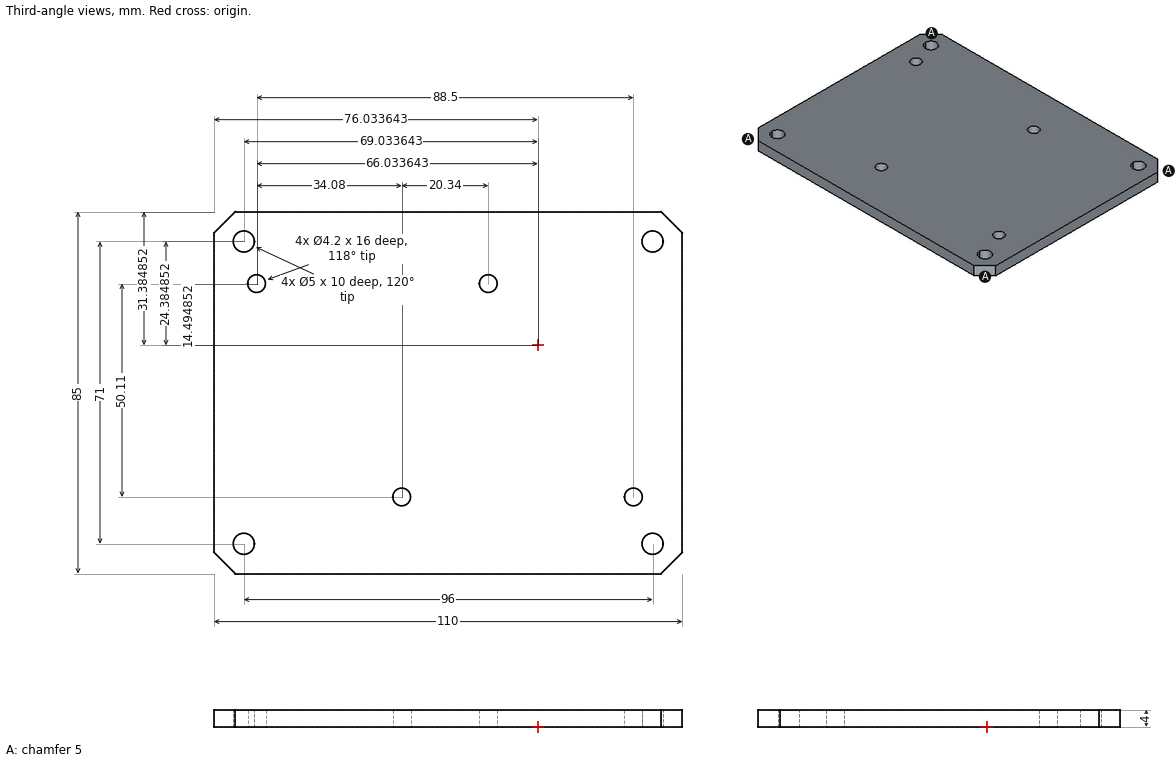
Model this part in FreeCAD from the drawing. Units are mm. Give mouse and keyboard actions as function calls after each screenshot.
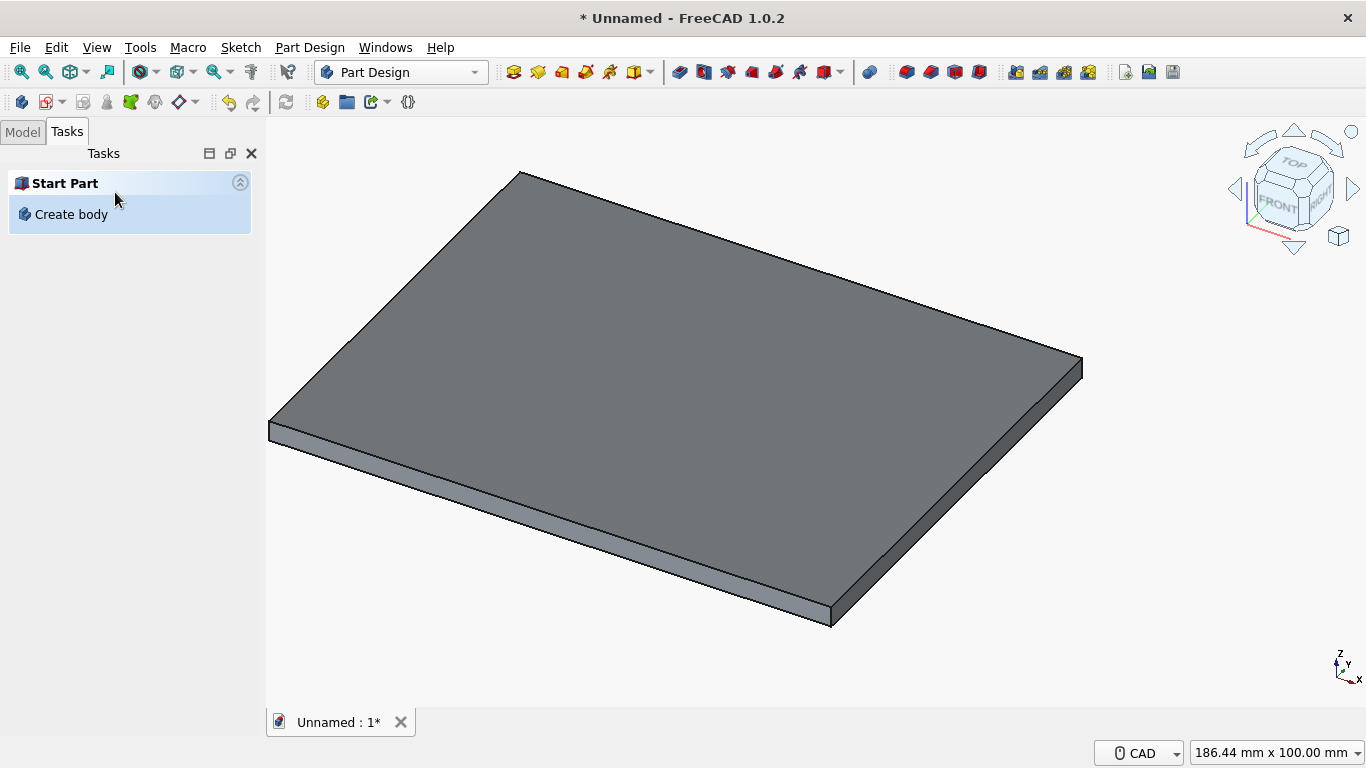
click(676, 389)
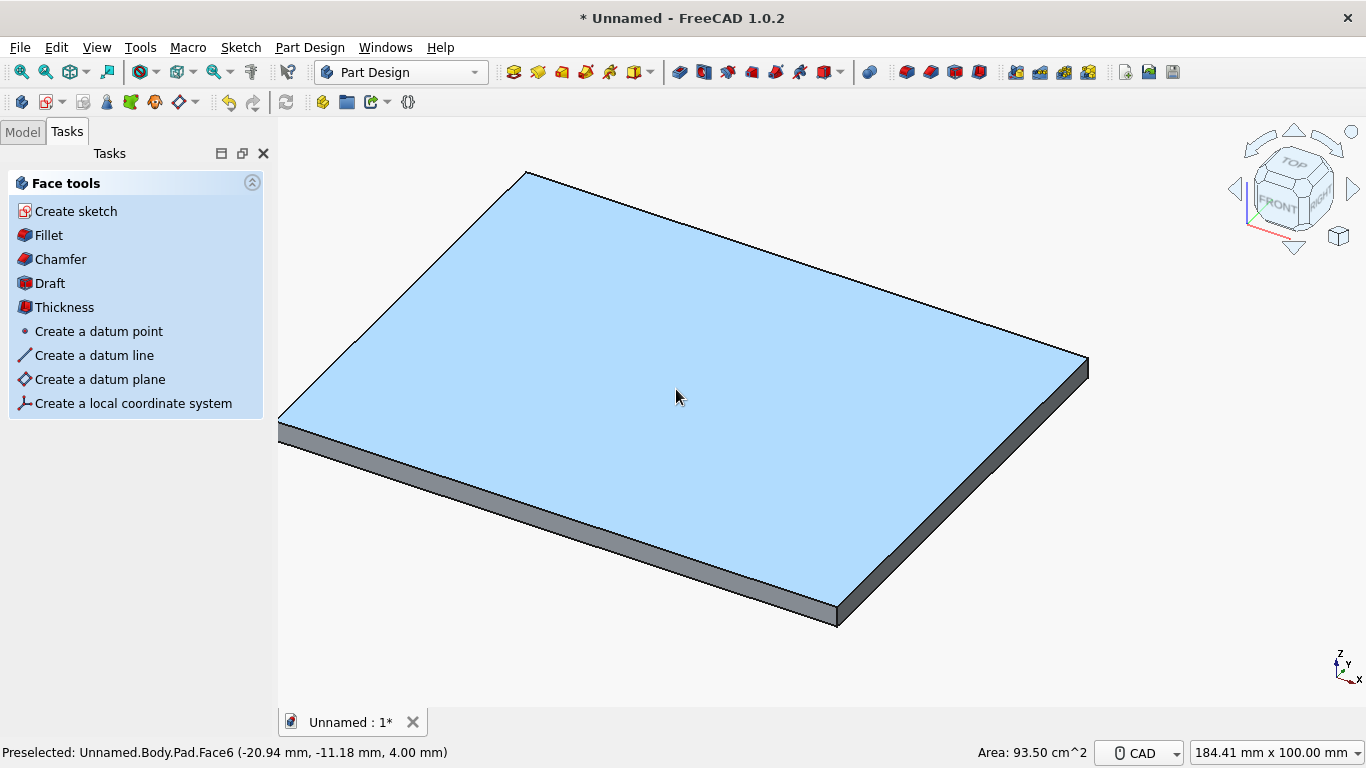
click(46, 102)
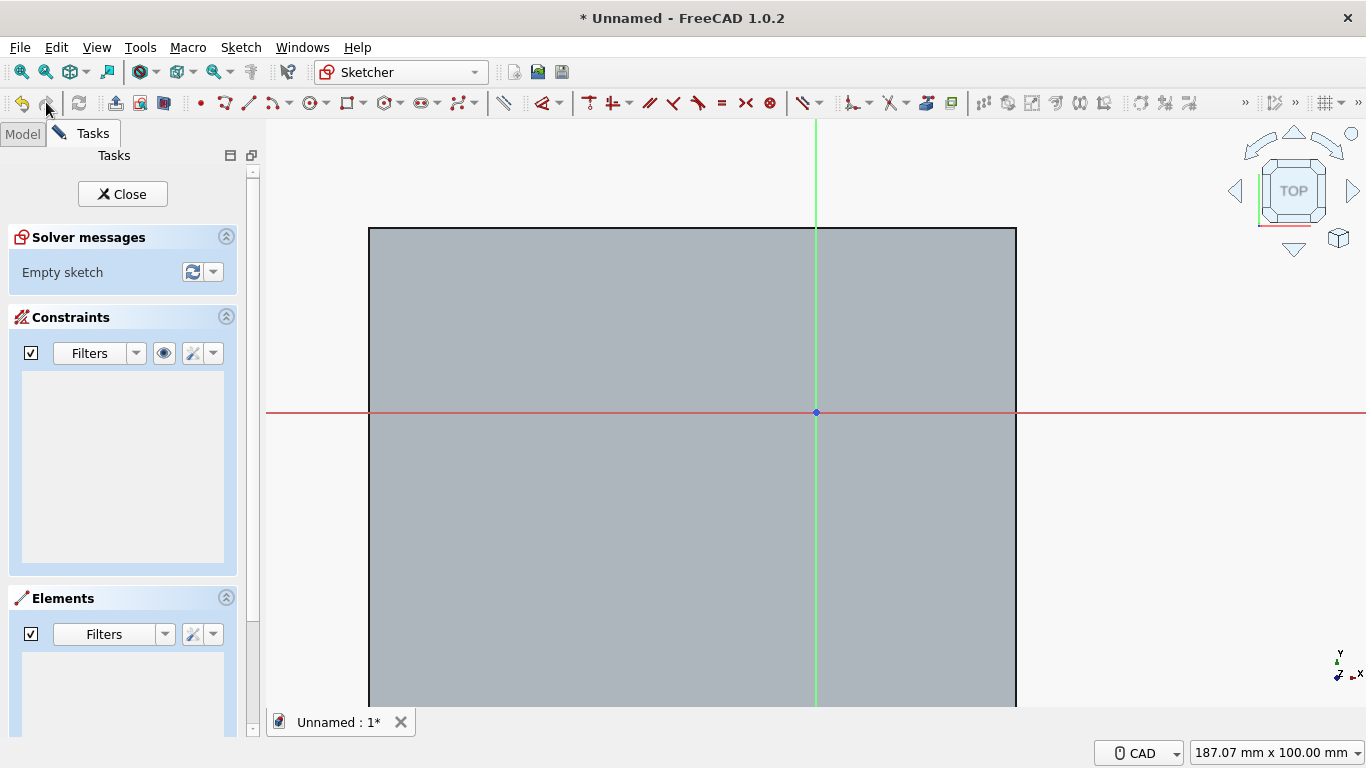
click(310, 104)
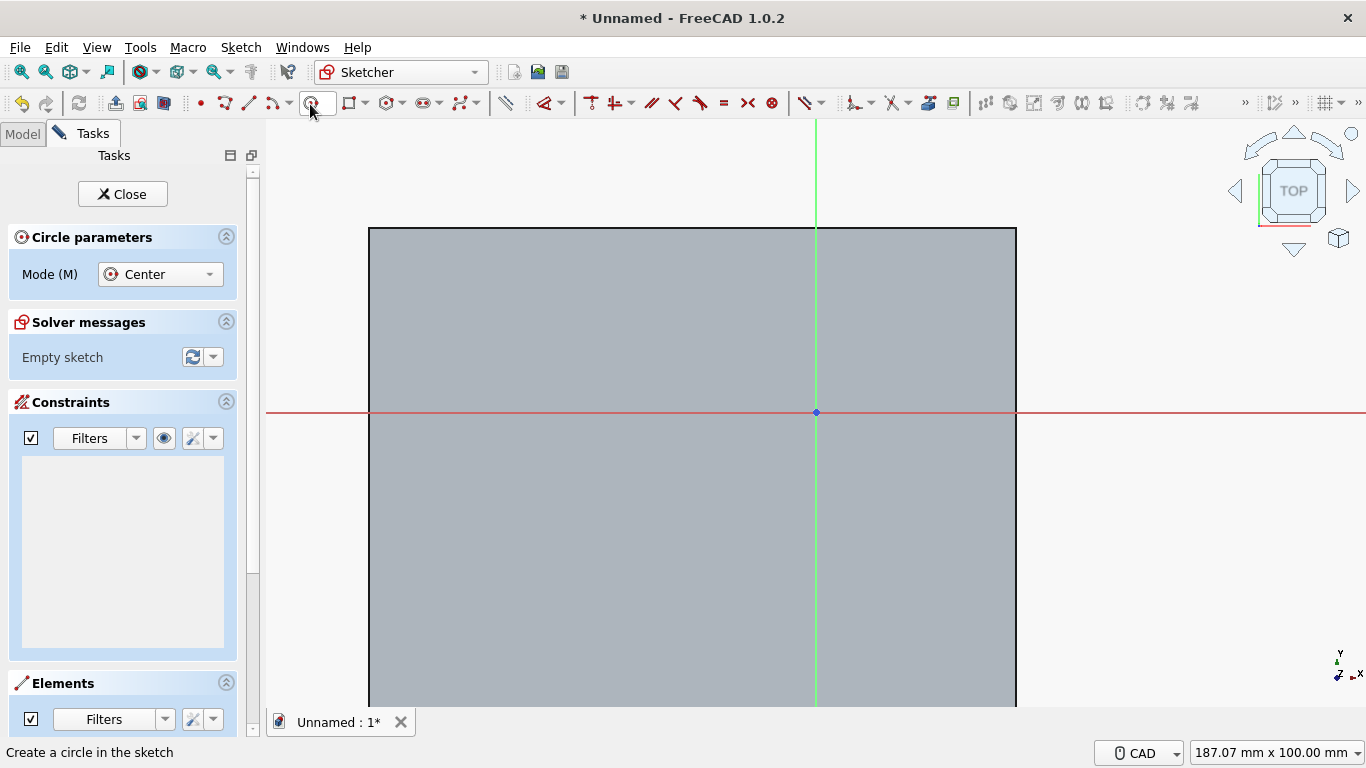
scroll(428, 328, up, 4)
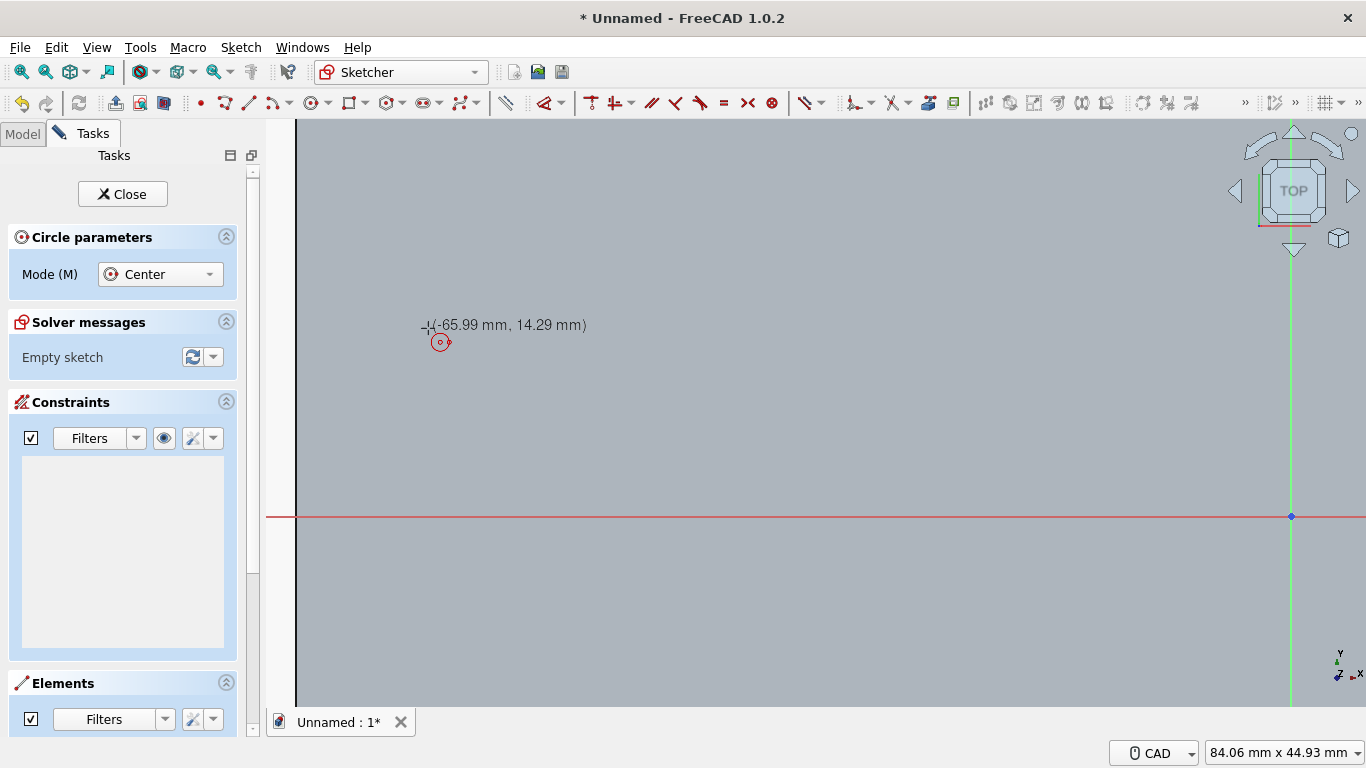
click(427, 327)
click(447, 308)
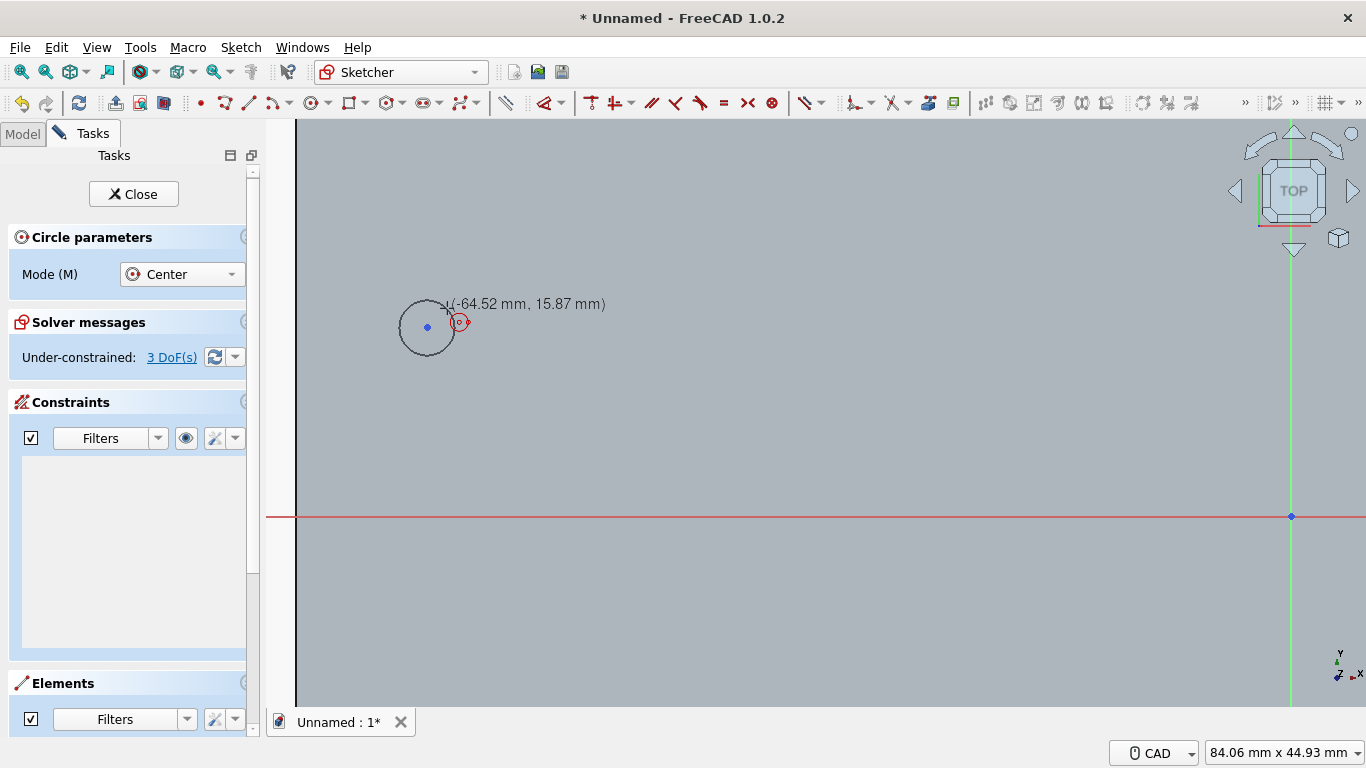
scroll(433, 147, down, 3)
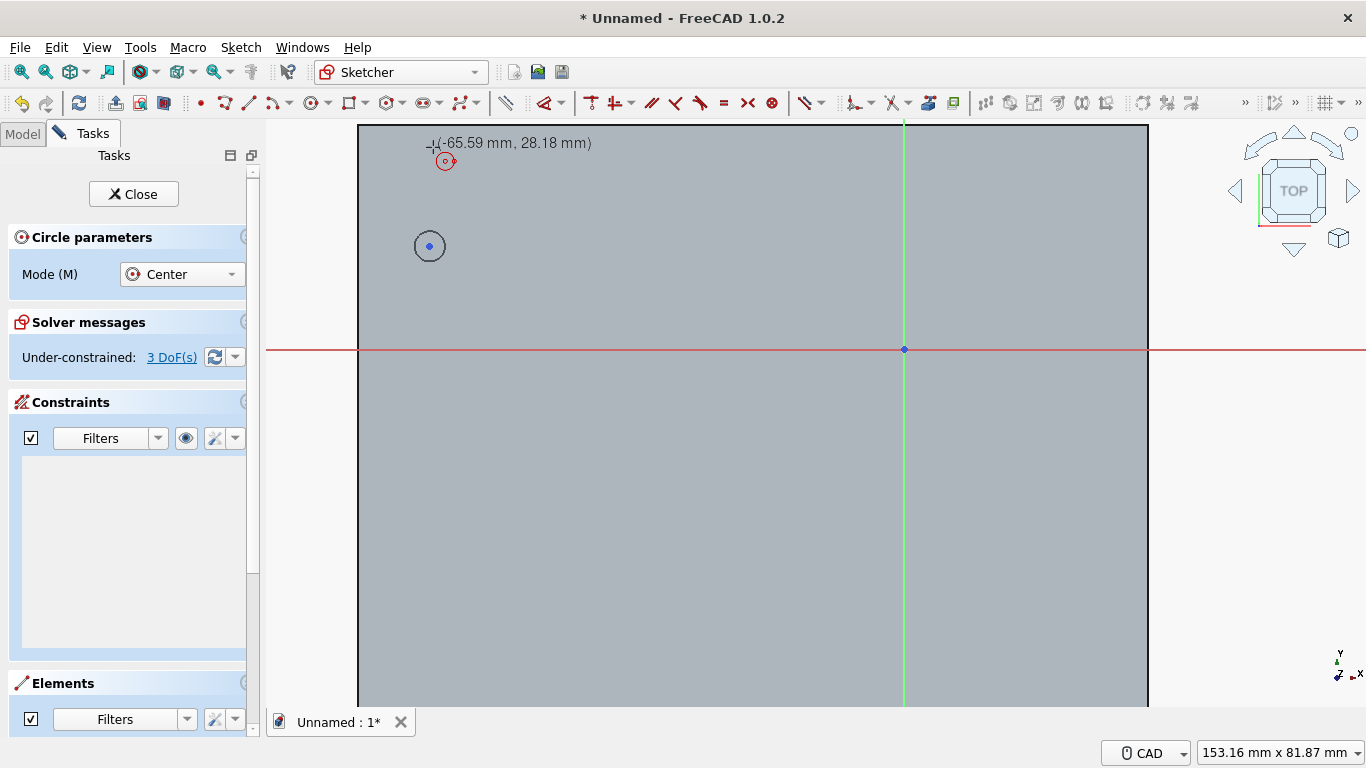
scroll(675, 606, up, 3)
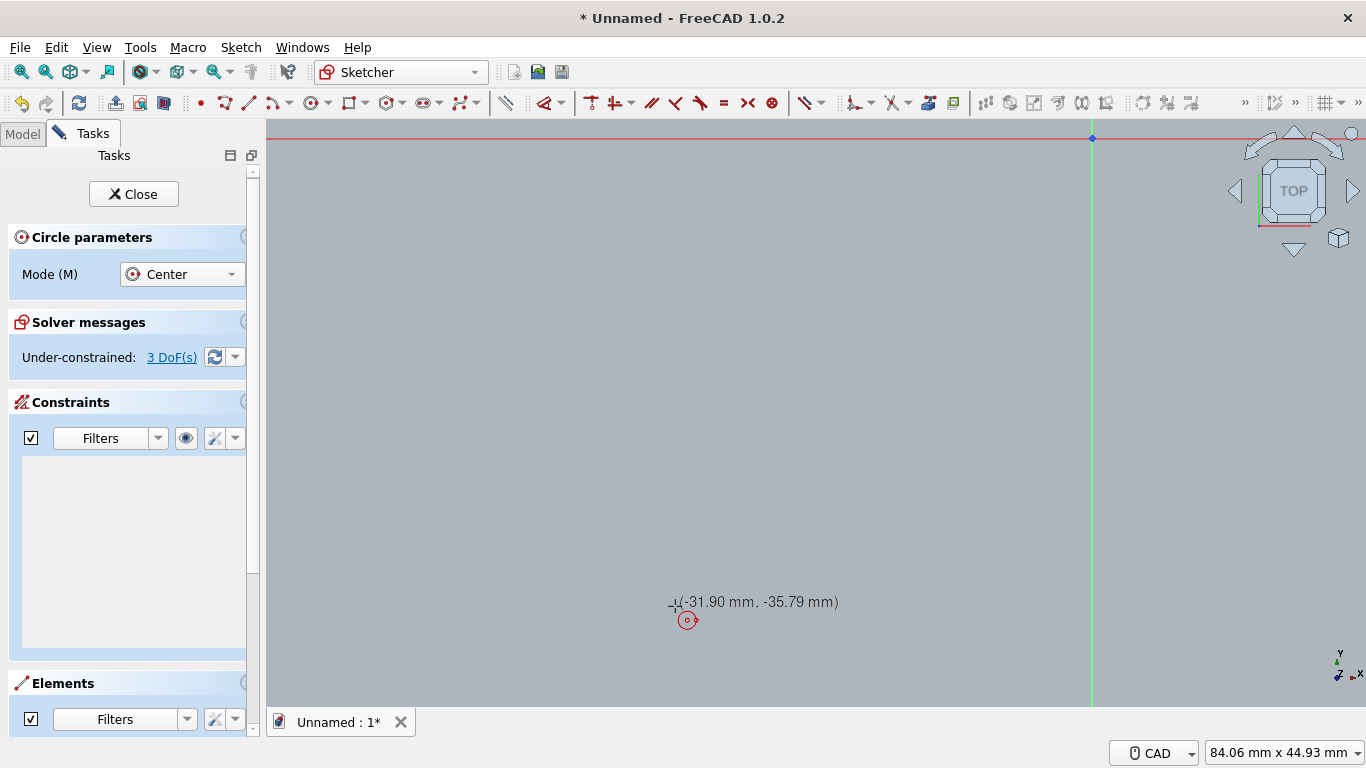
click(674, 605)
click(693, 585)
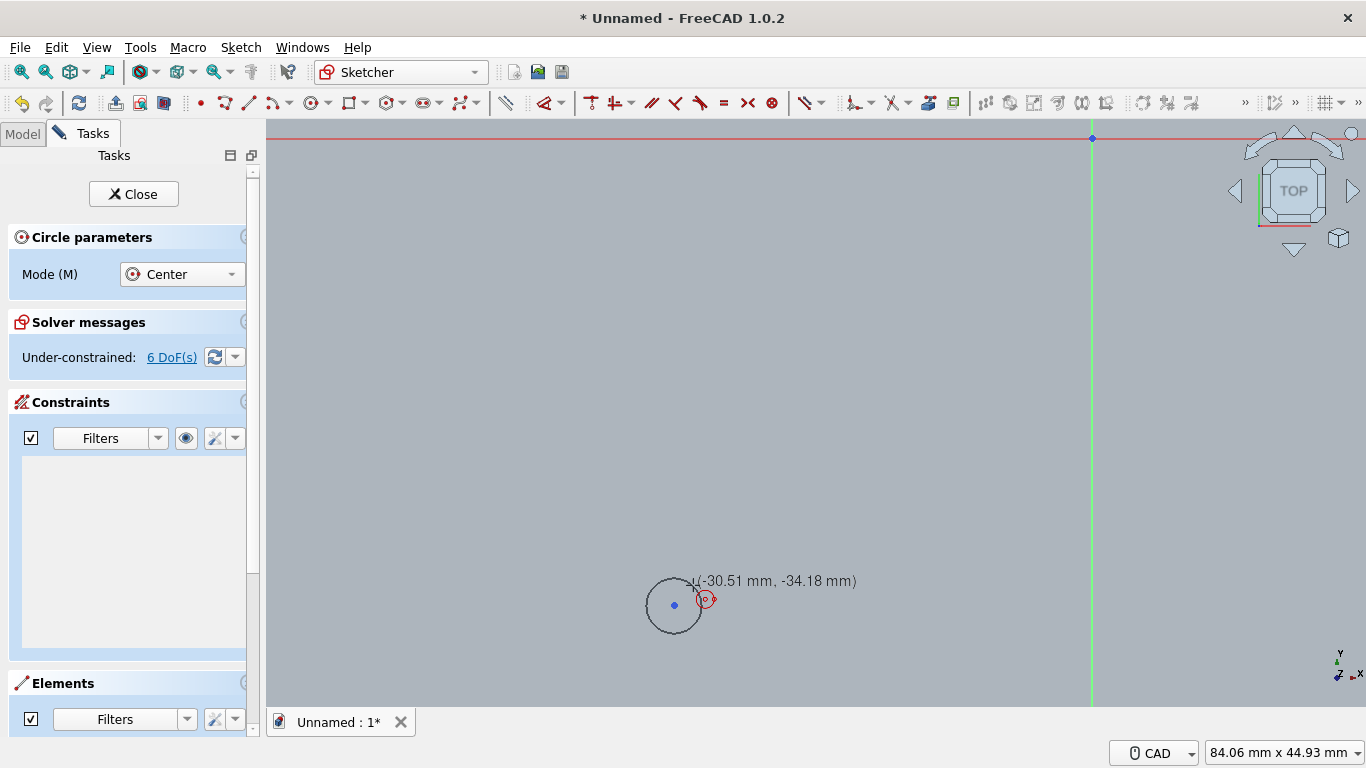
scroll(675, 579, down, 3)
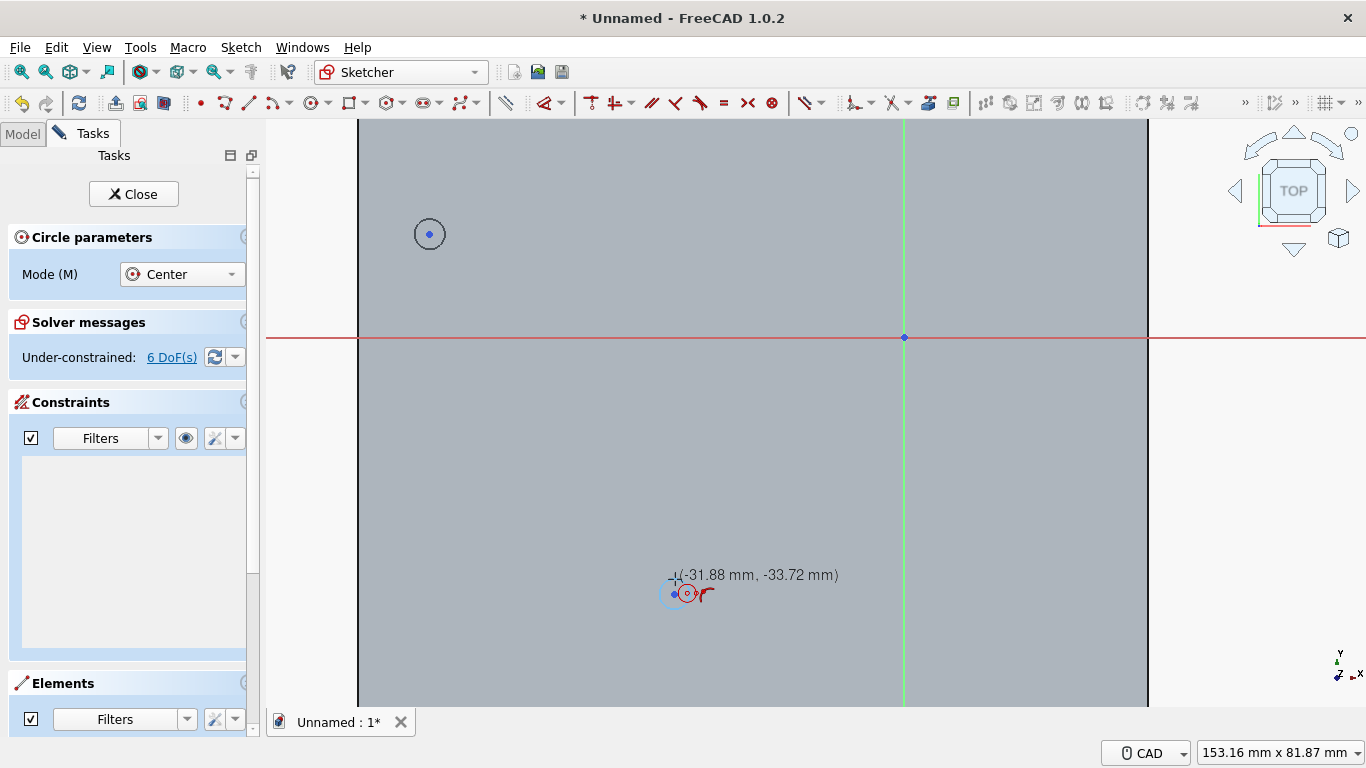
scroll(821, 234, up, 3)